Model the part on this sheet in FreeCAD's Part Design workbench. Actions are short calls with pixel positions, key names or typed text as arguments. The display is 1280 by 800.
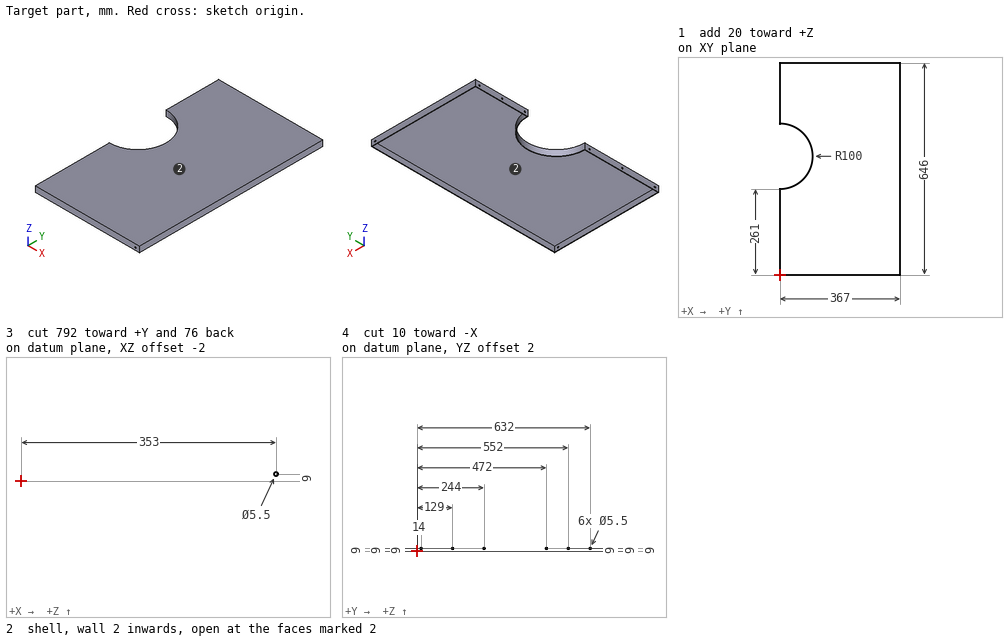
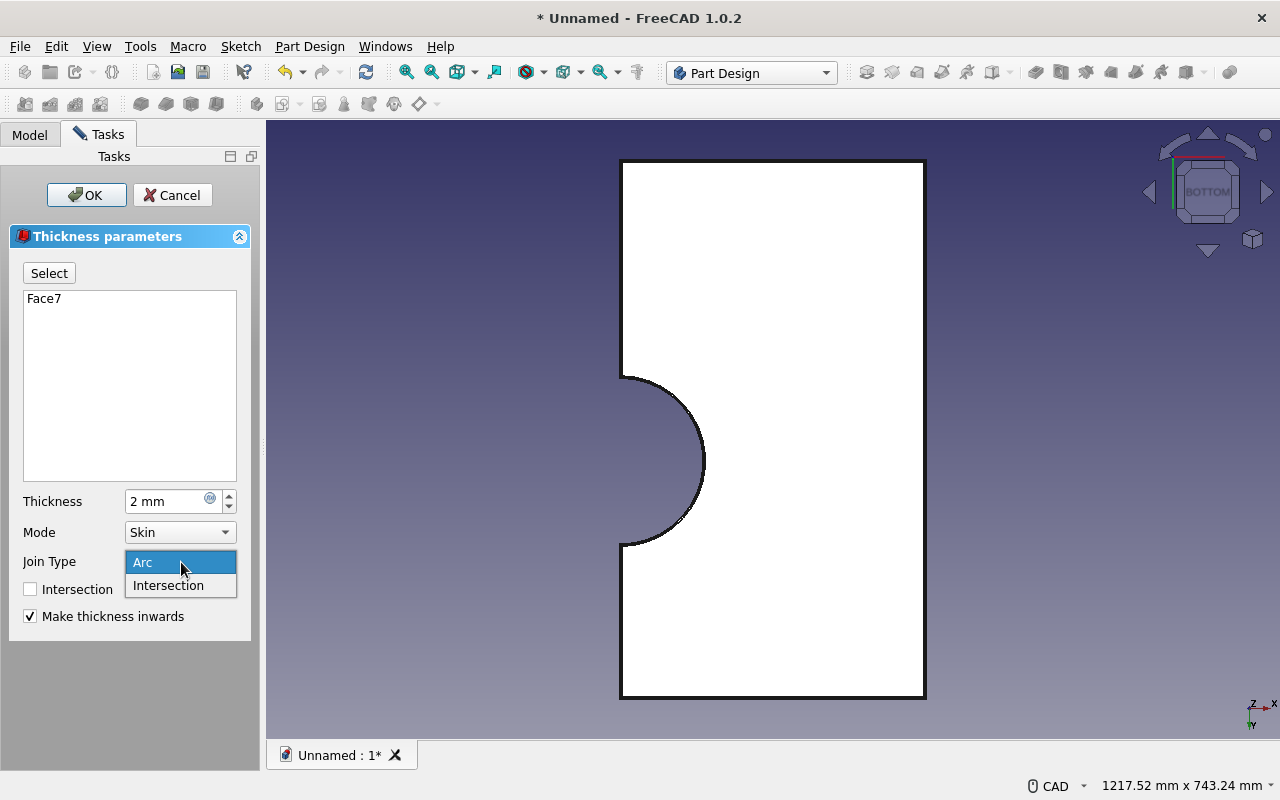
click(179, 586)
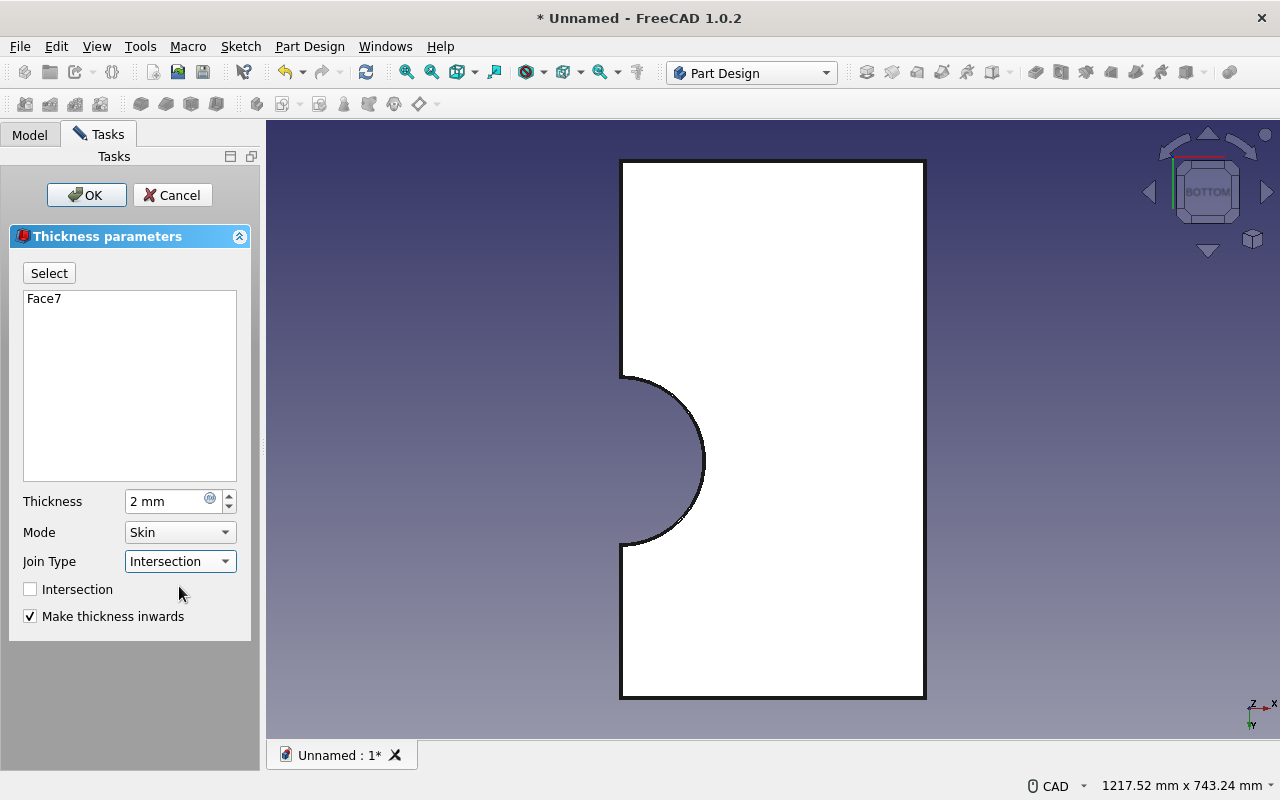
click(87, 195)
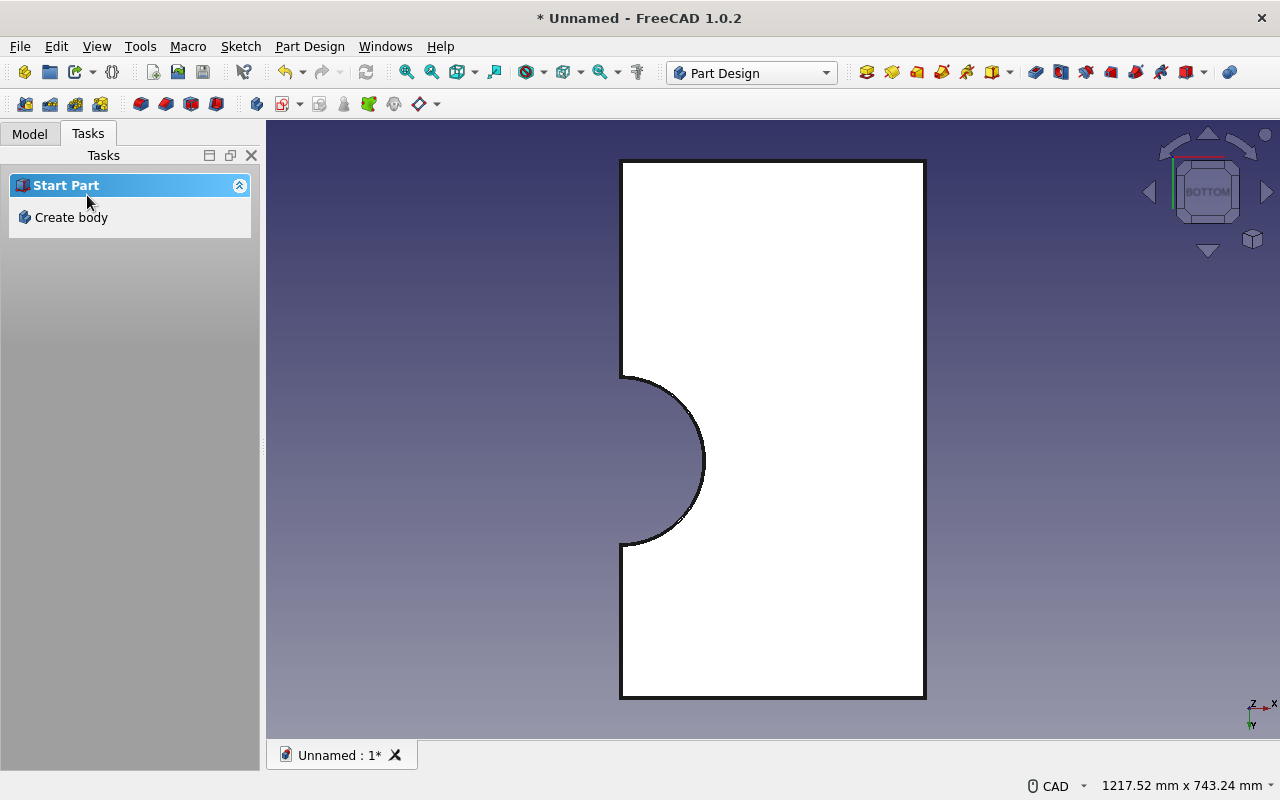
click(30, 134)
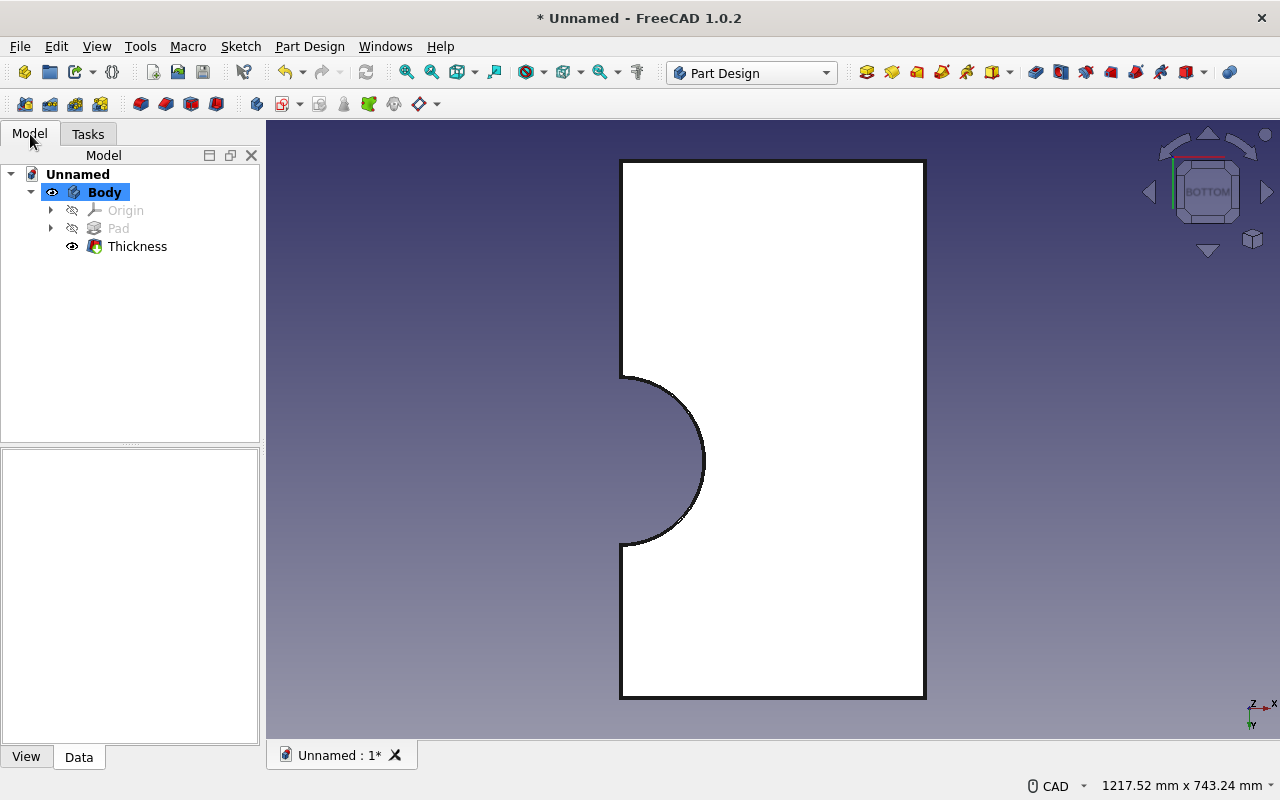
click(51, 210)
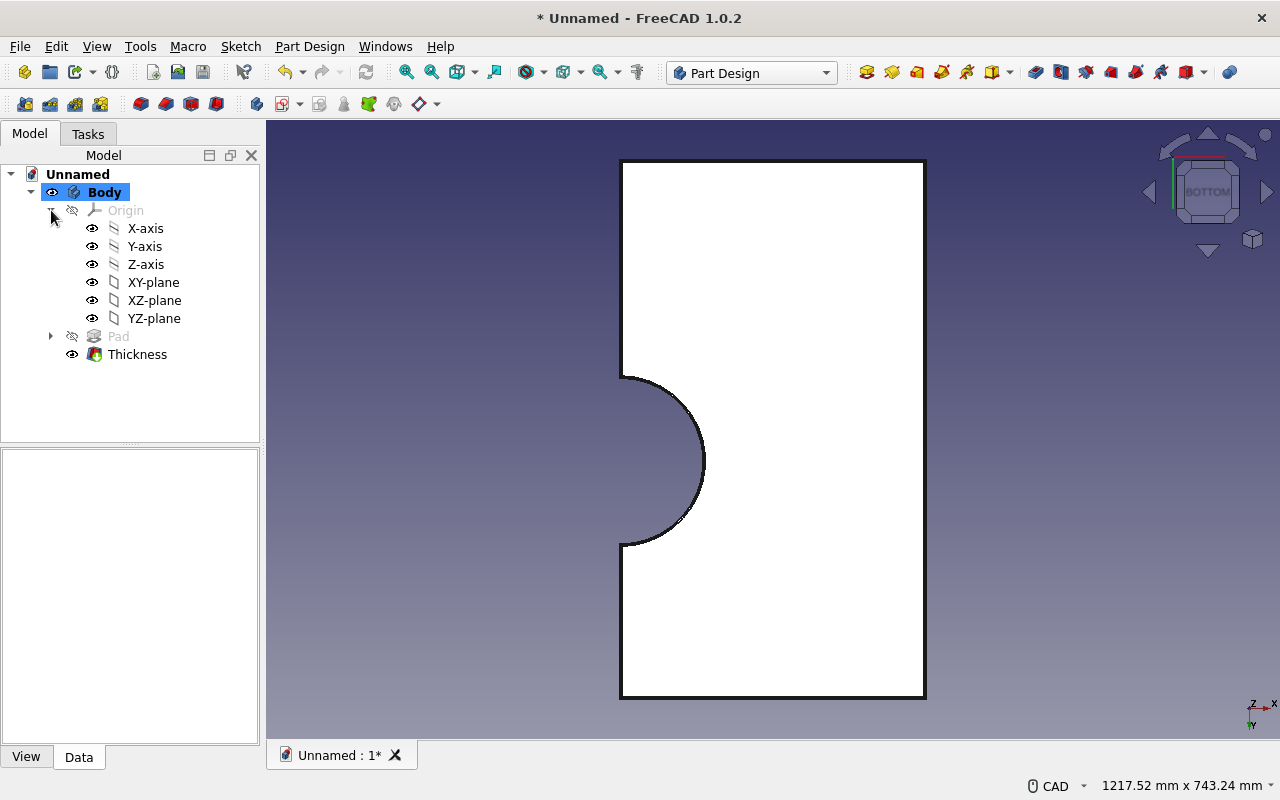
click(137, 300)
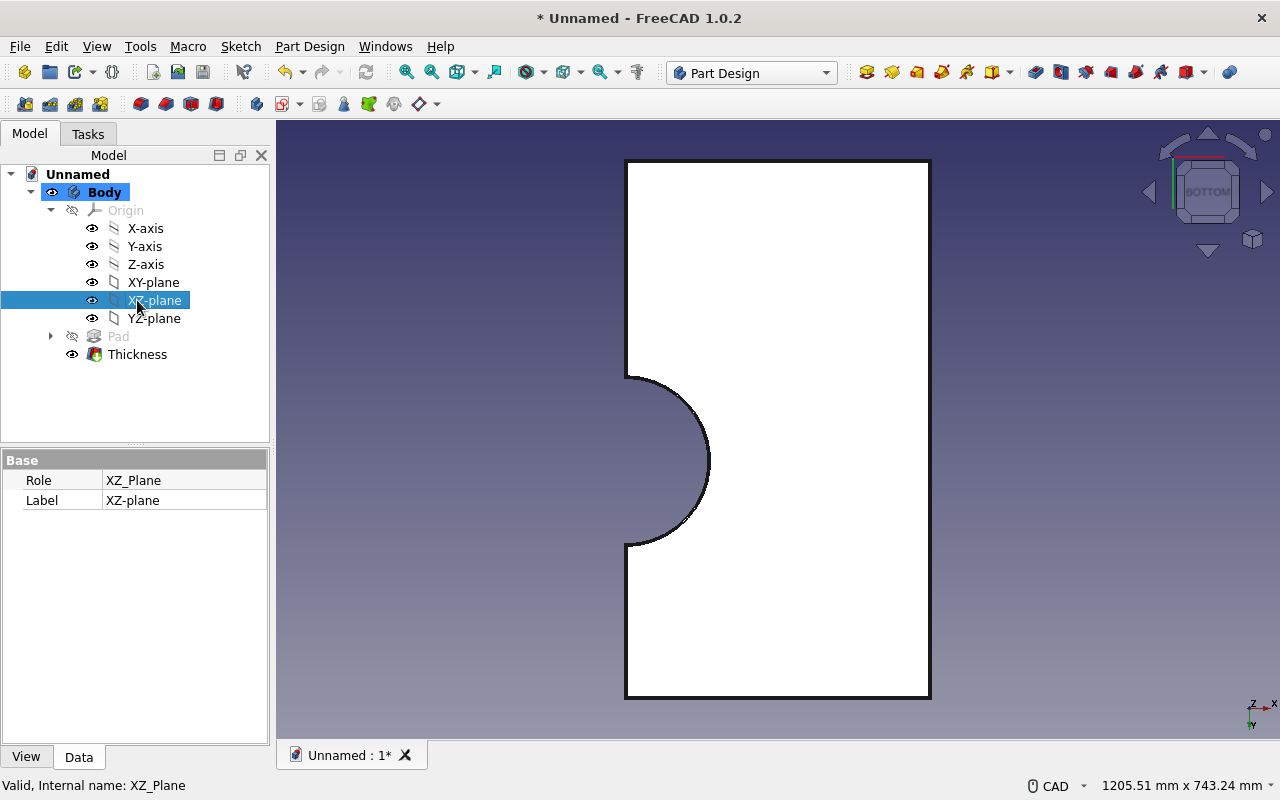
click(418, 104)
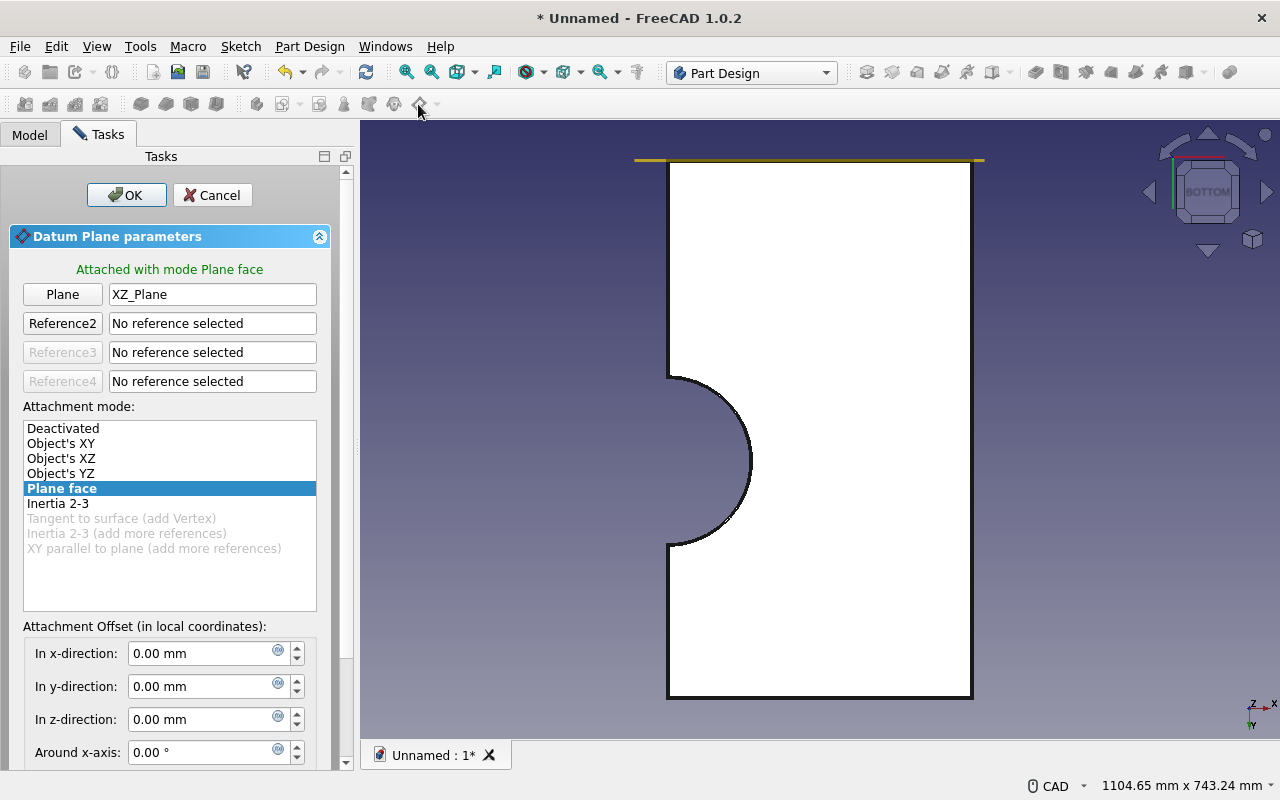
triple_click(210, 720)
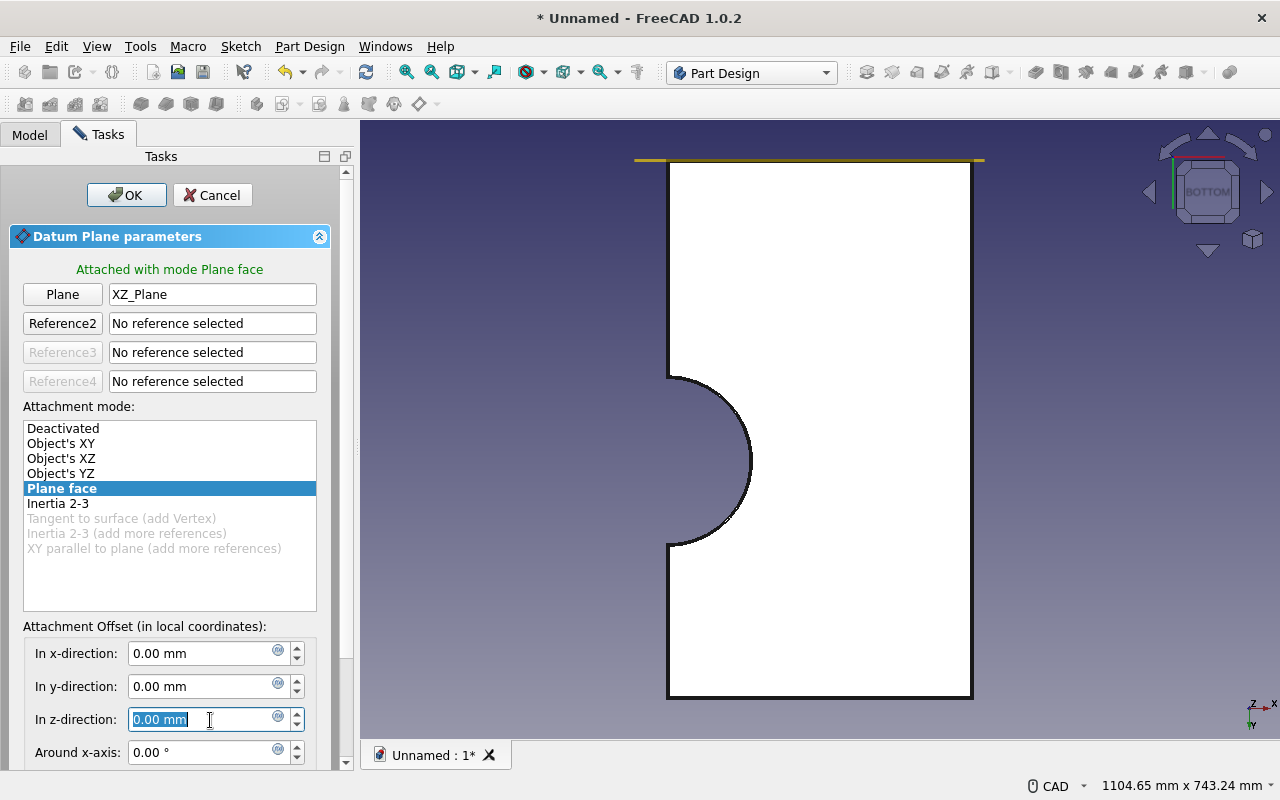
text(-2)
key(Tab)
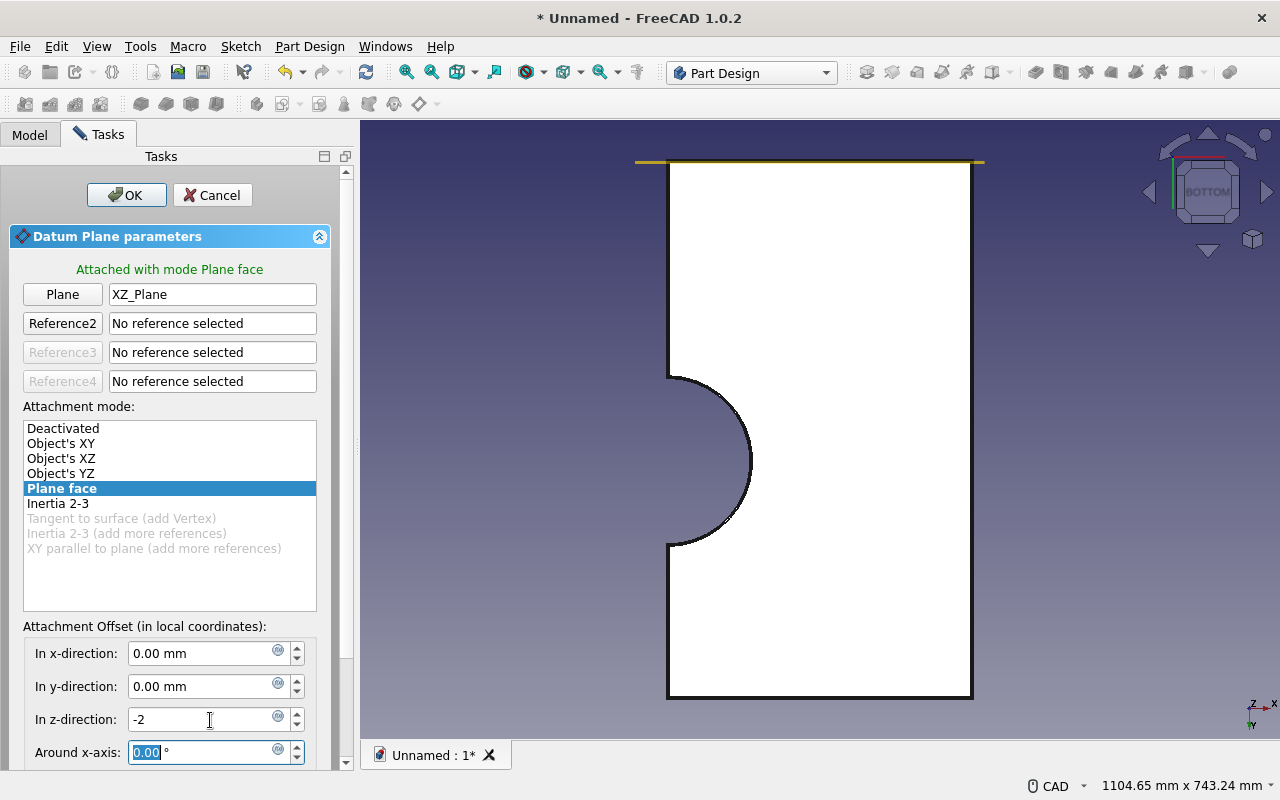
click(127, 195)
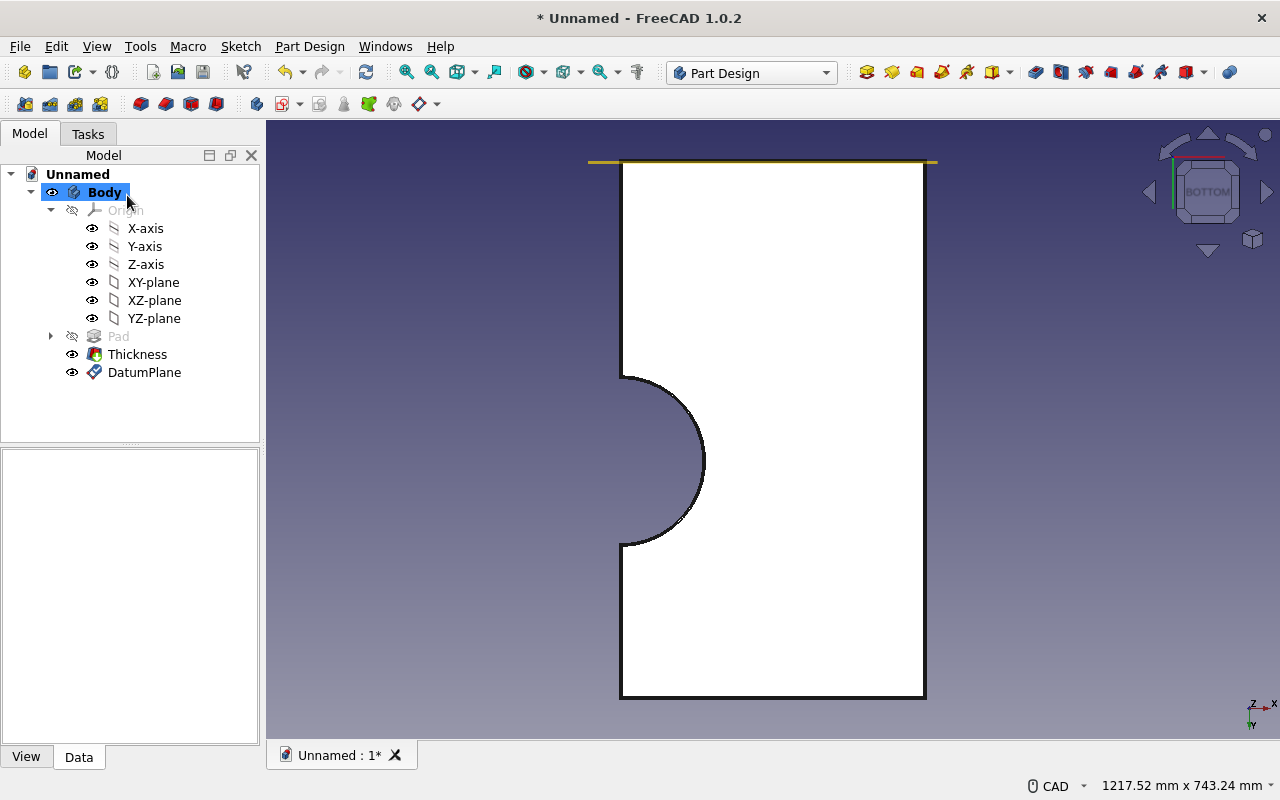
click(117, 372)